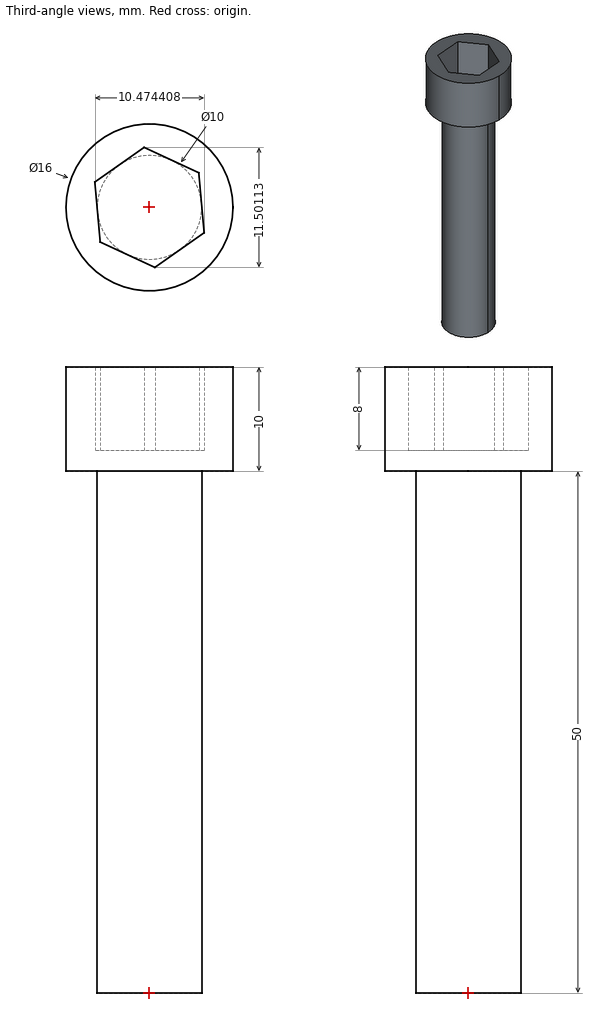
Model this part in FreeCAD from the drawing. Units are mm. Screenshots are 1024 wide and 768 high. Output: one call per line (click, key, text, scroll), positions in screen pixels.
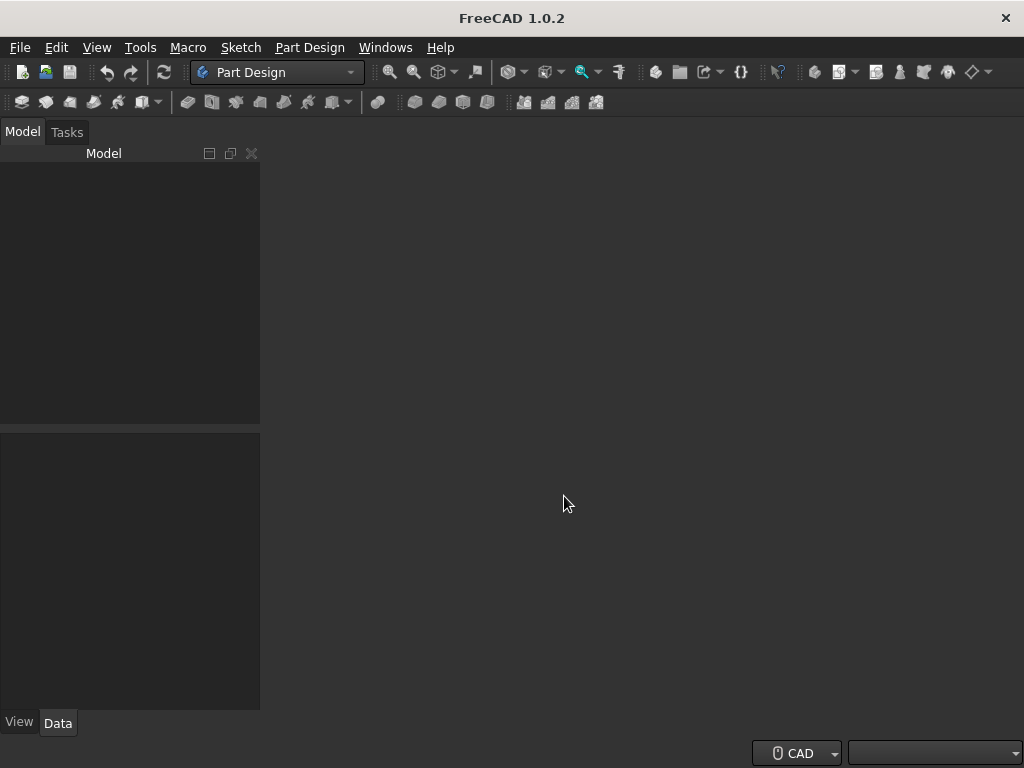
key(ctrl+n)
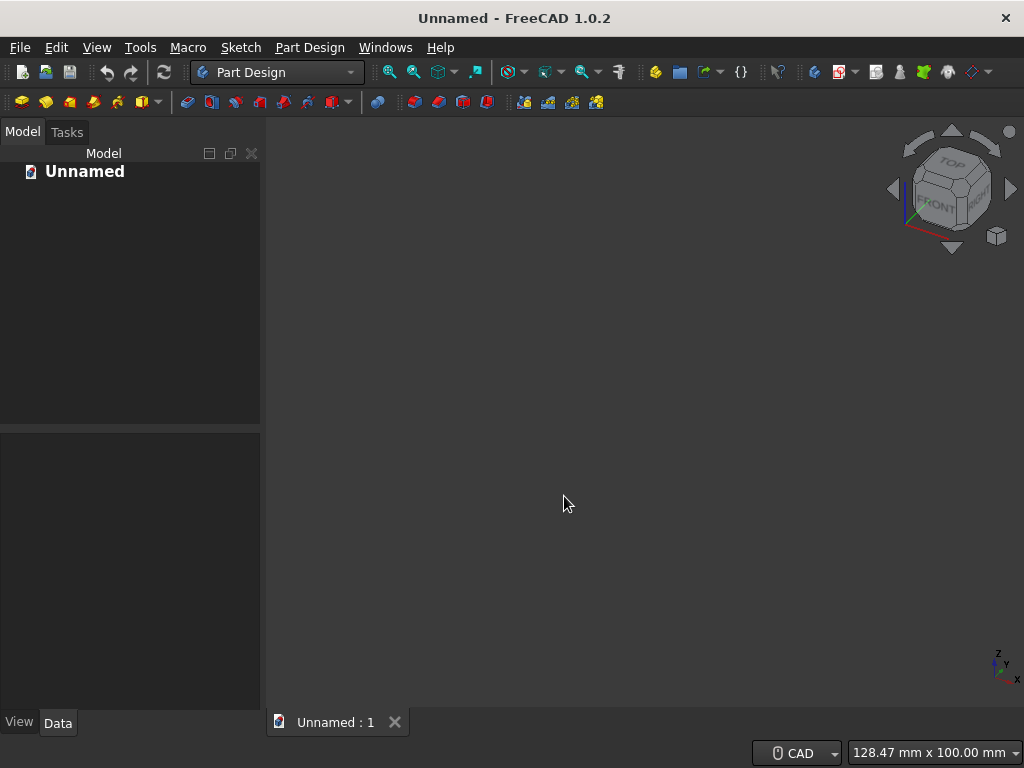
click(840, 72)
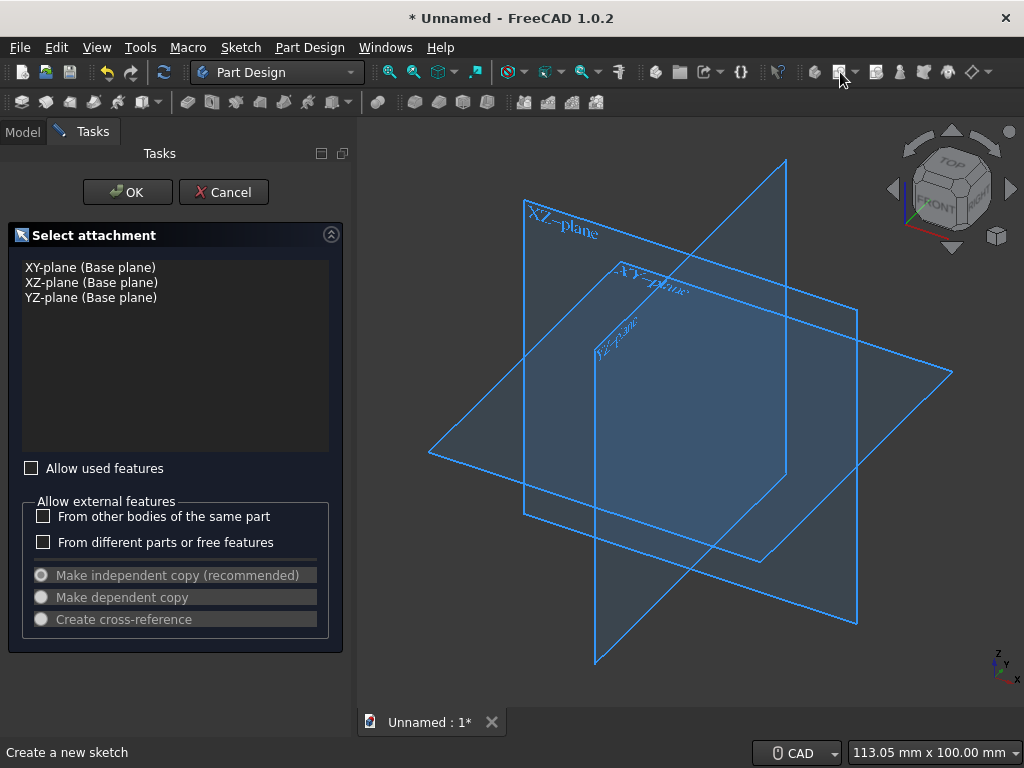
click(82, 268)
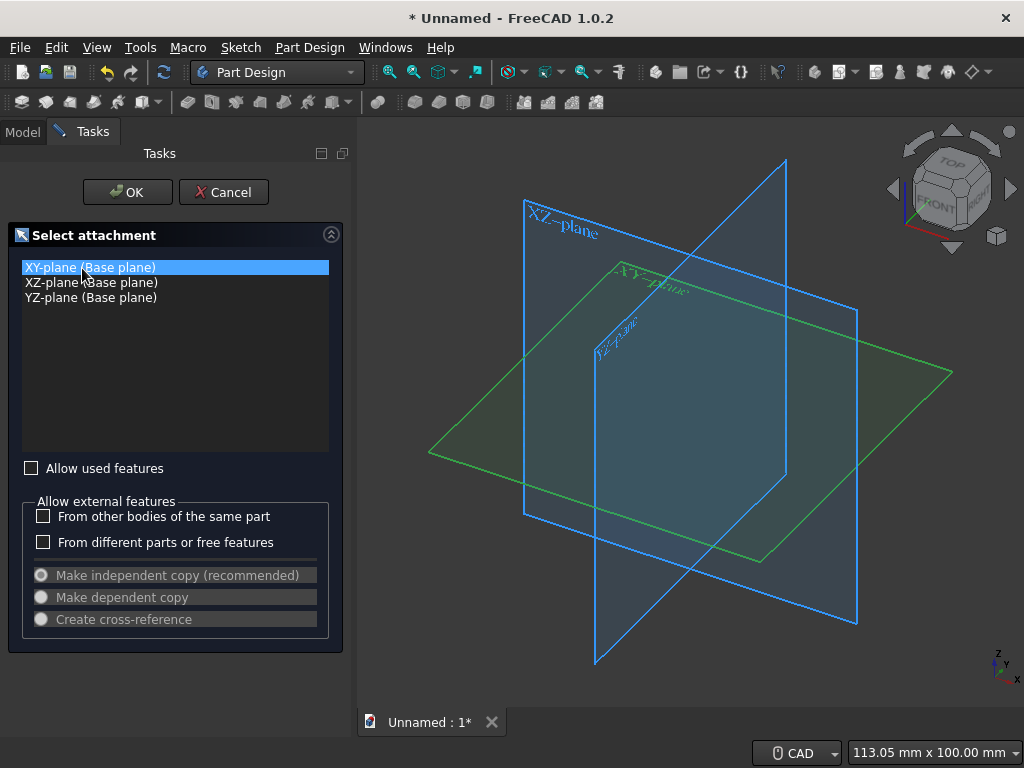
click(128, 192)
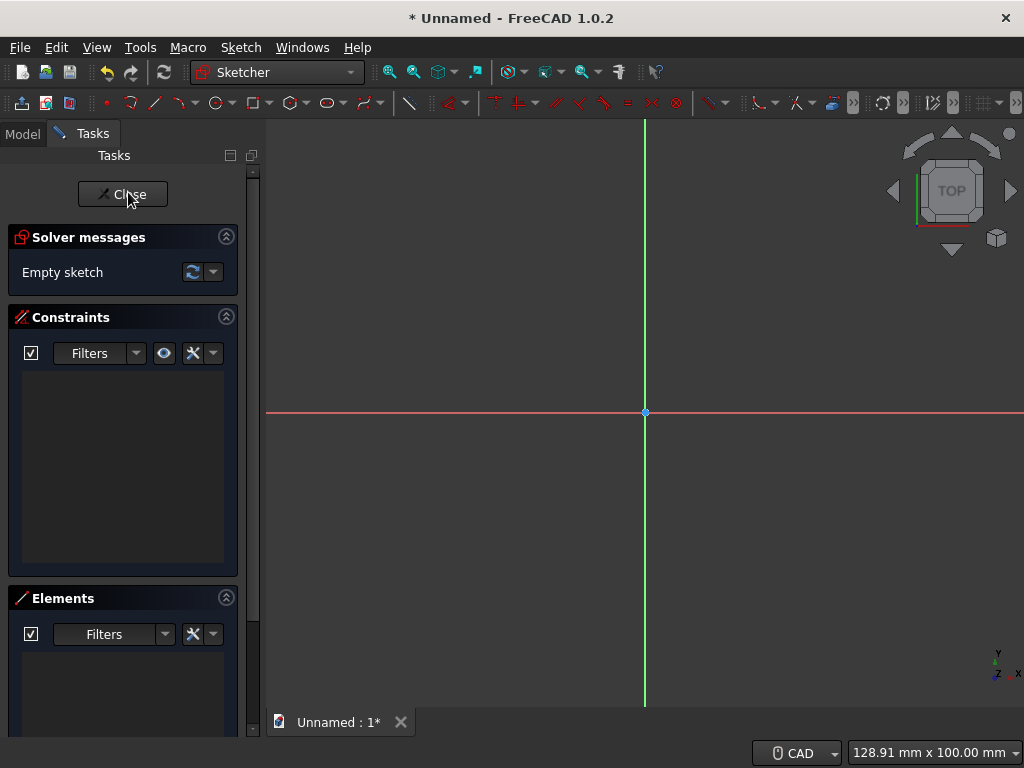
scroll(659, 413, up, 9)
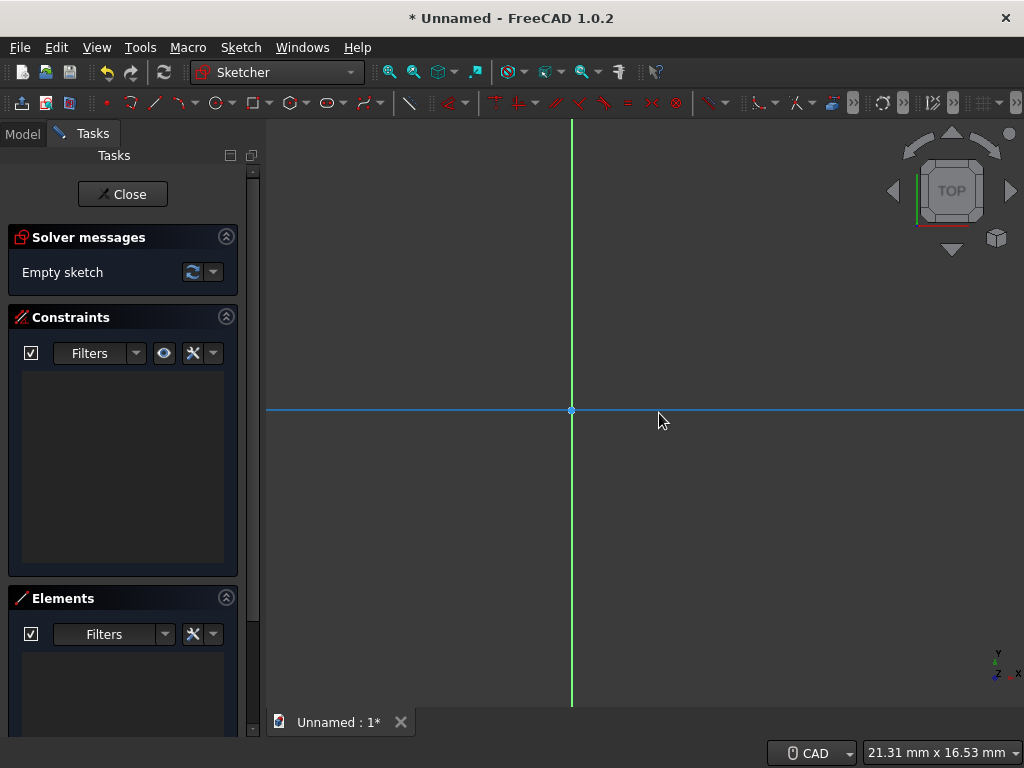
key(g)
key(c)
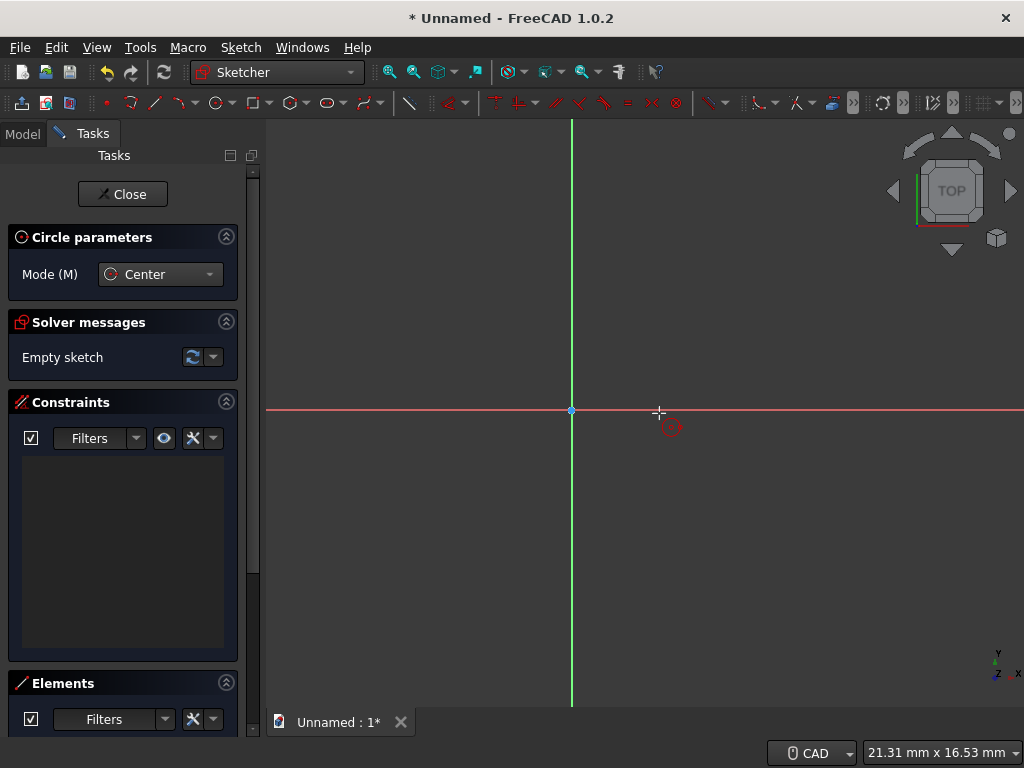
click(572, 410)
click(697, 285)
key(Escape)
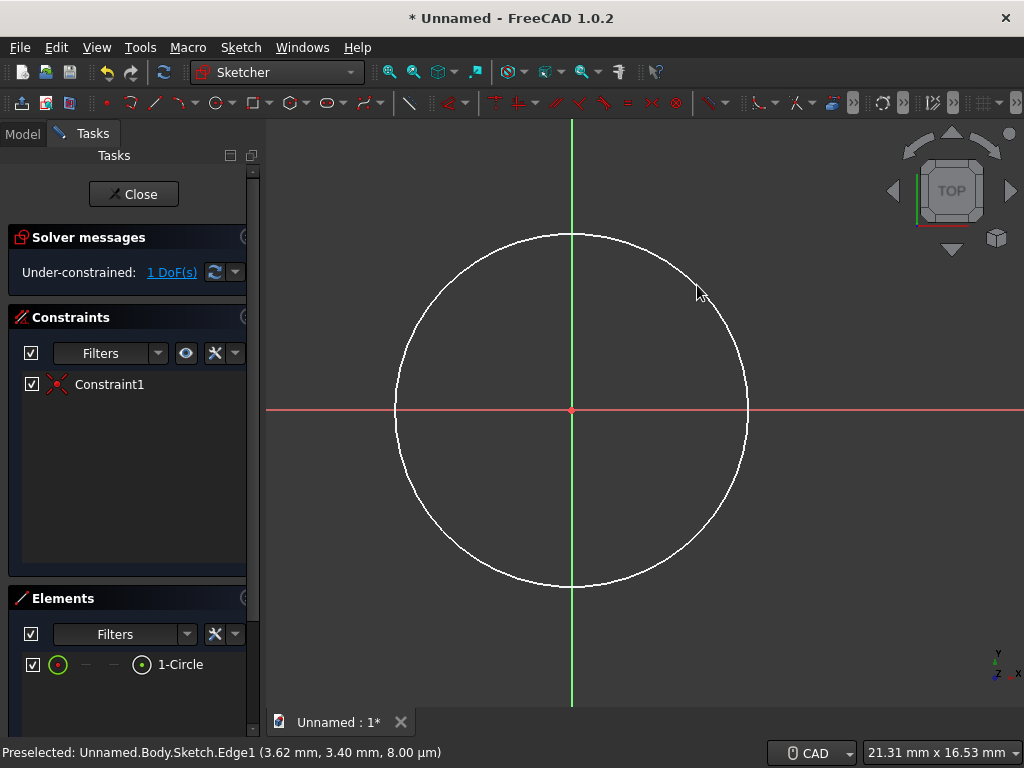
click(696, 285)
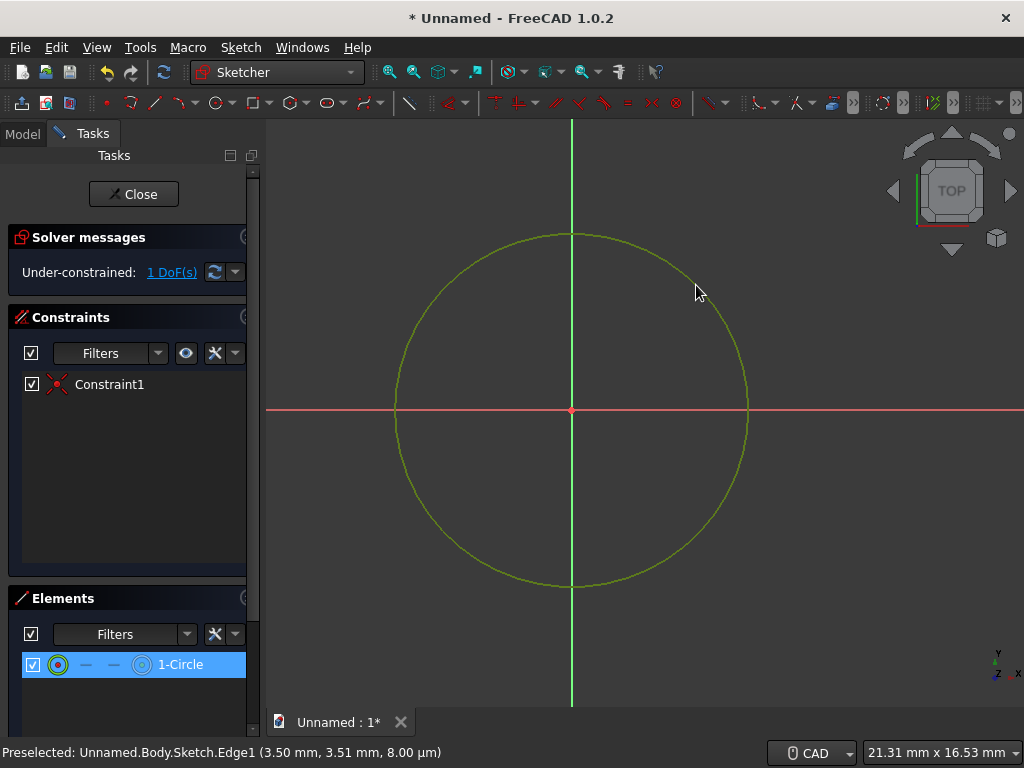
key(k)
key(o)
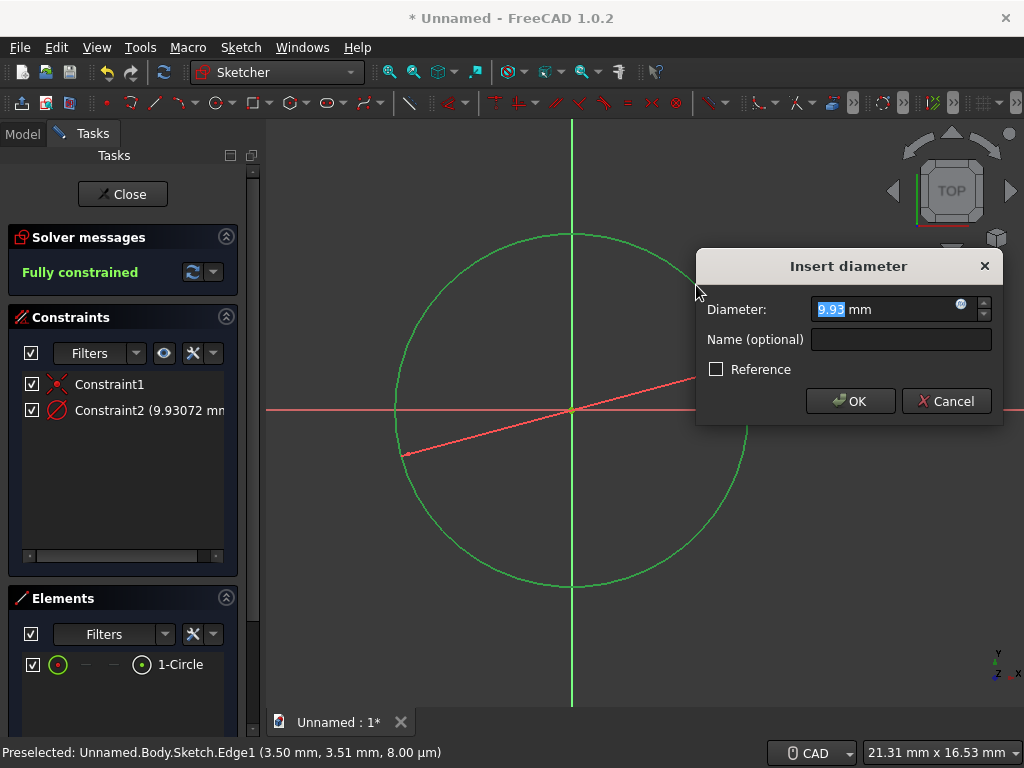
text(10)
key(Return)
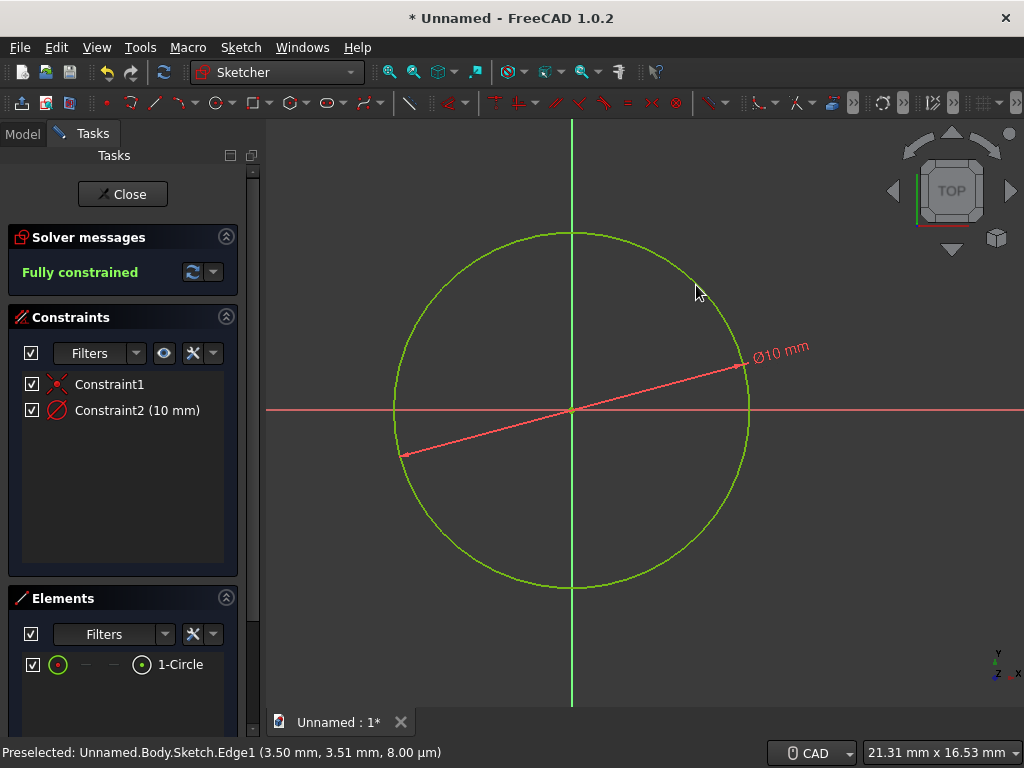
click(123, 194)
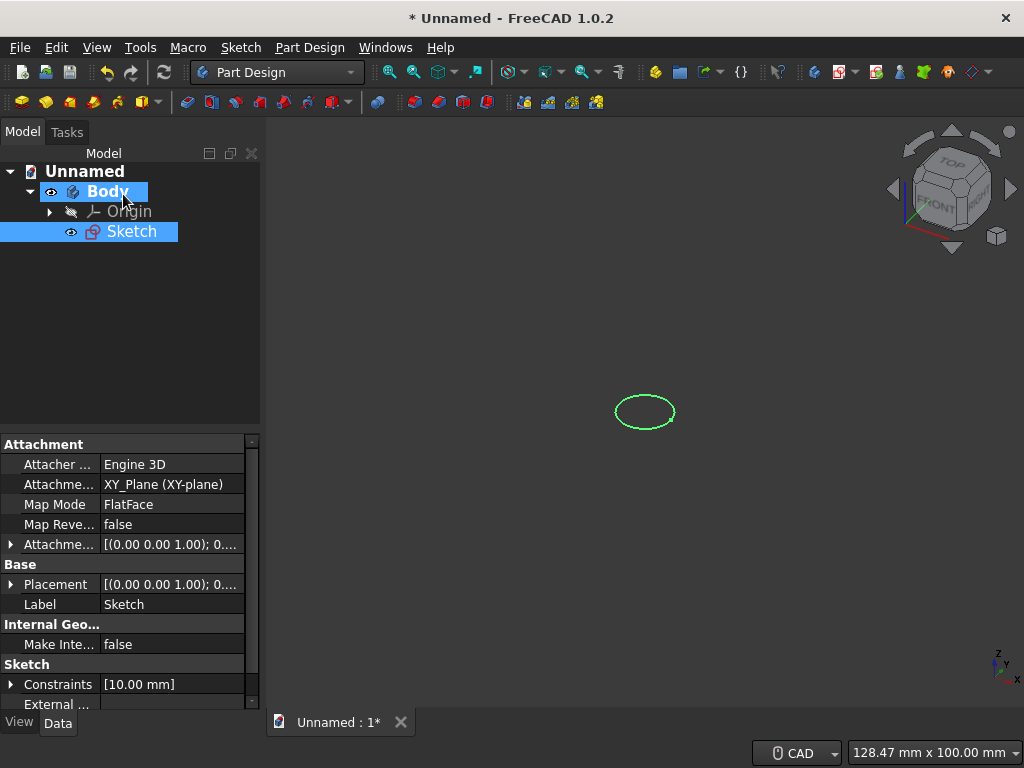
click(22, 102)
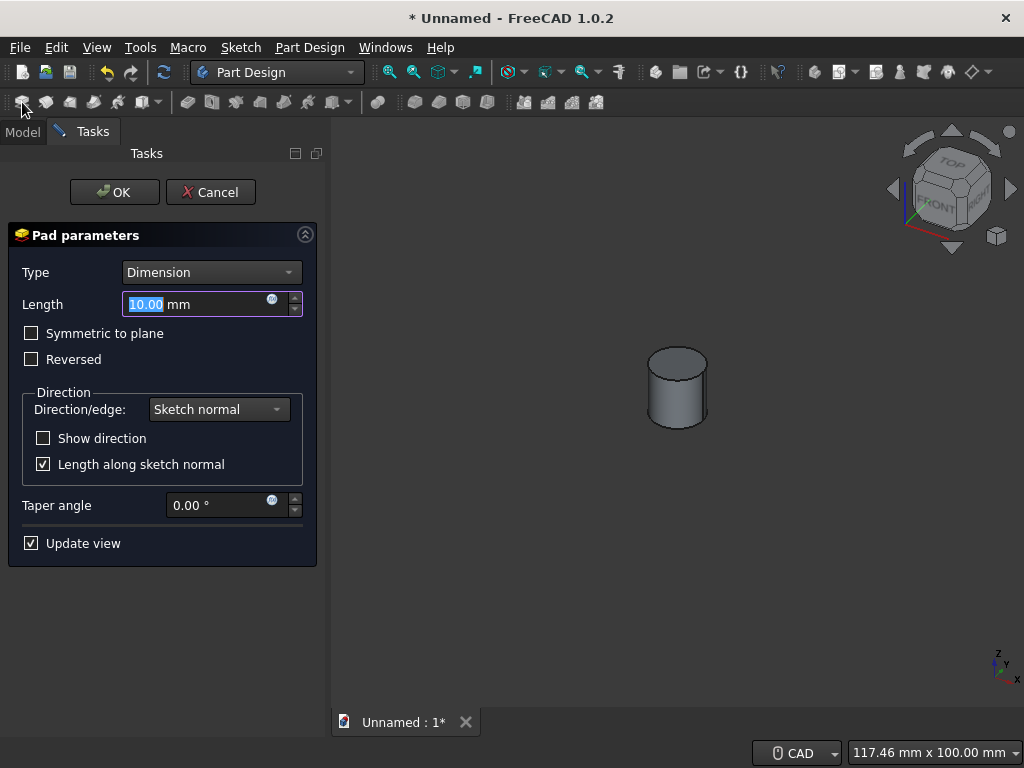
text(50)
key(Tab)